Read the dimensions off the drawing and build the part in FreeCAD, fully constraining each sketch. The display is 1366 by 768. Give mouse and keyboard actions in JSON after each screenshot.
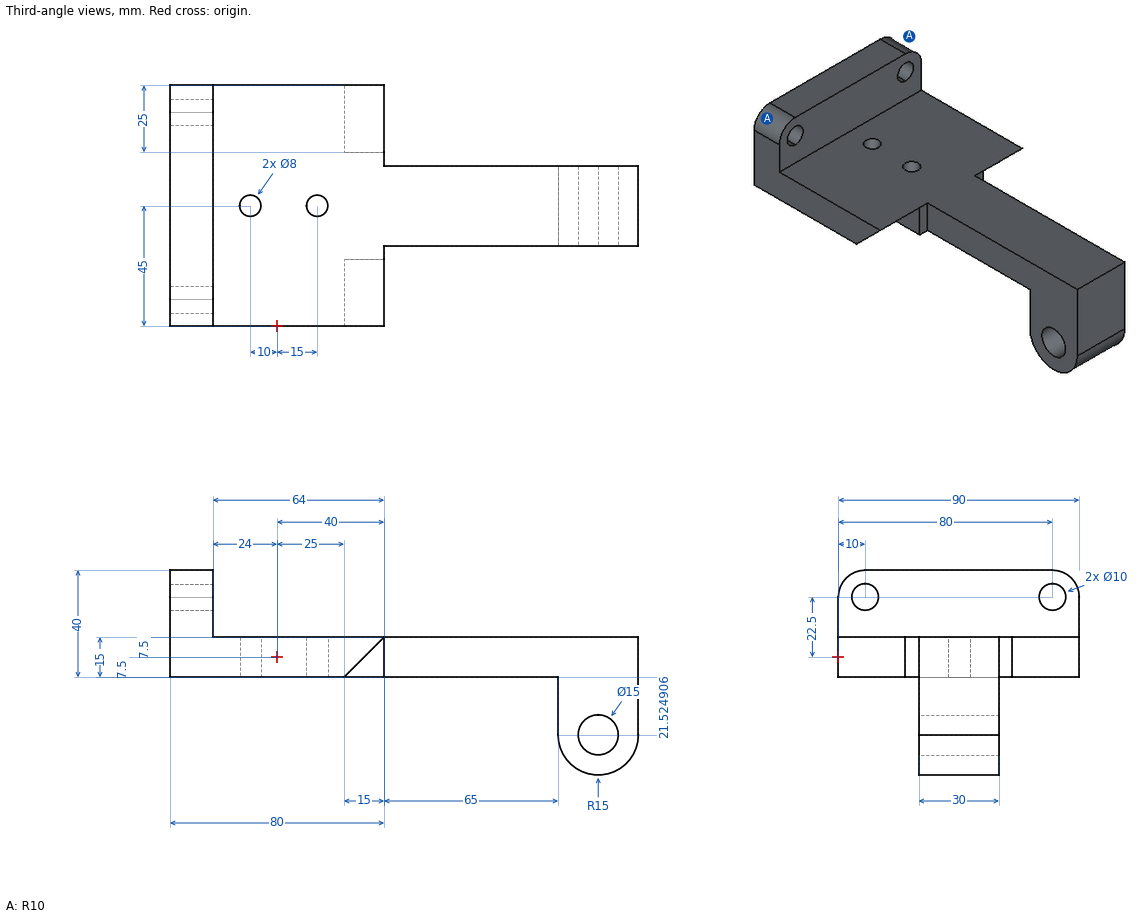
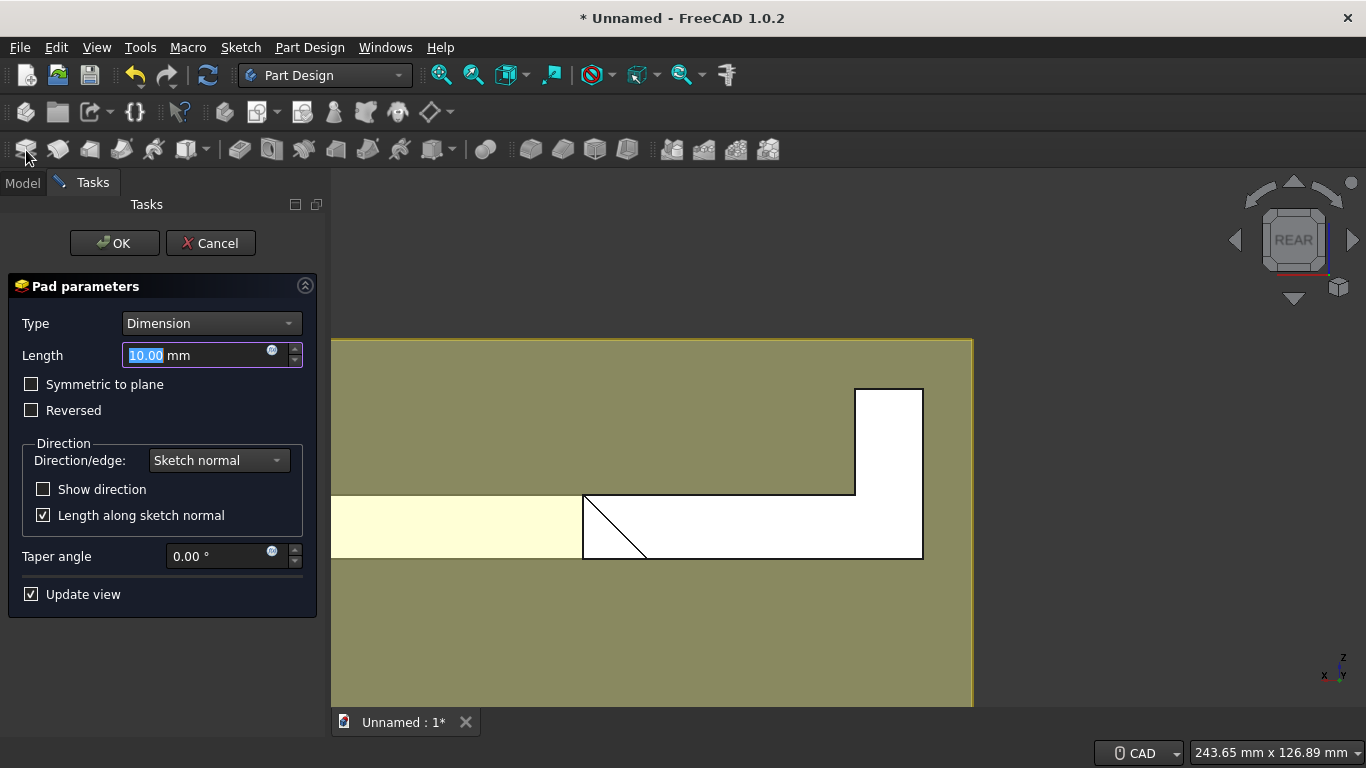
{"action": "type", "text": "30"}
{"action": "key", "text": "Tab"}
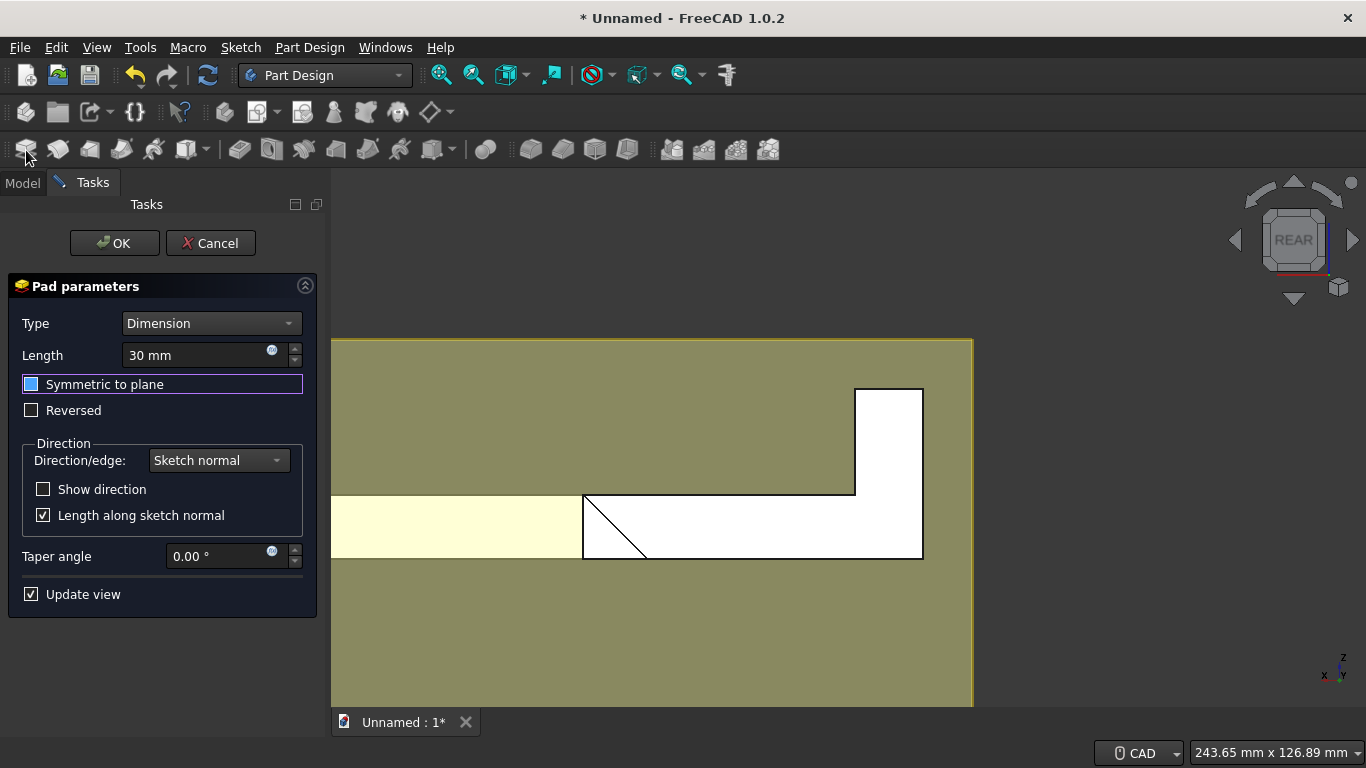
{"action": "left_click", "coordinate": [30, 384]}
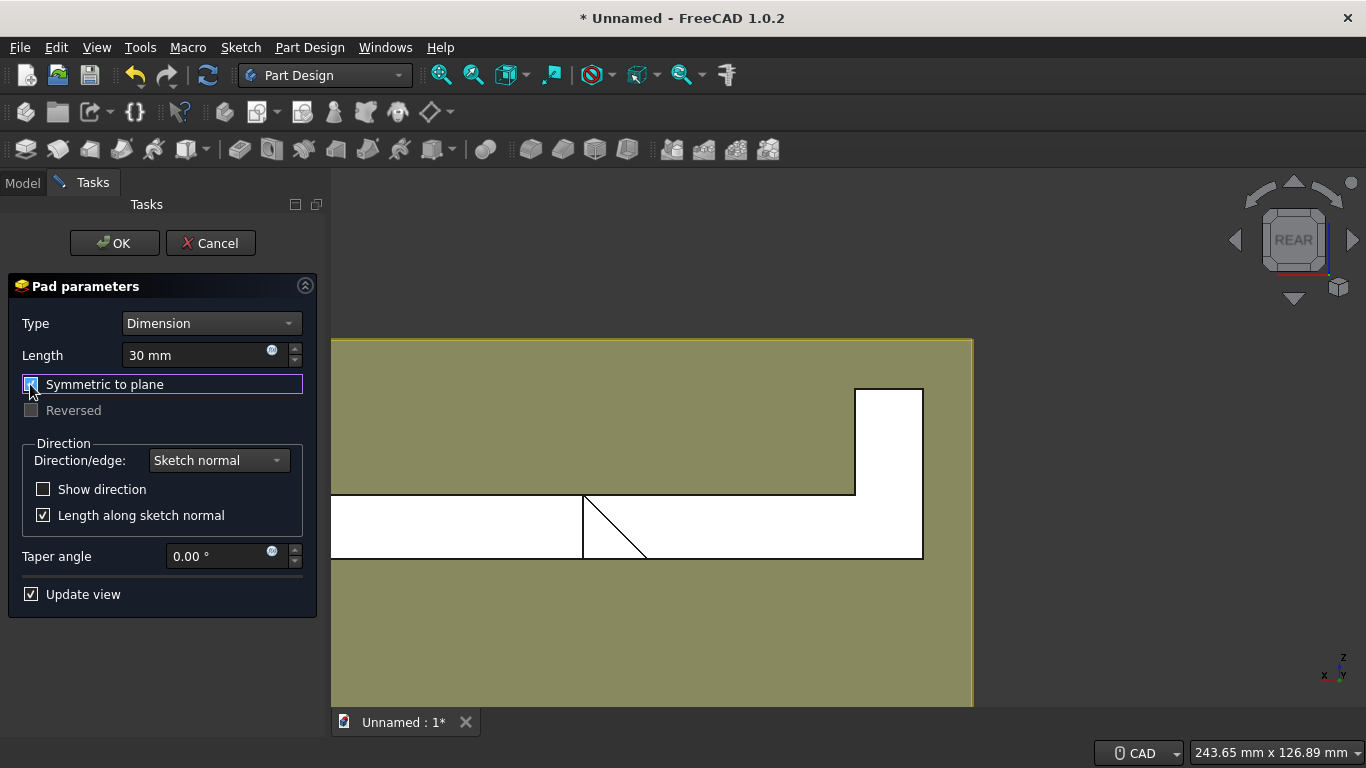
{"action": "left_click", "coordinate": [115, 243]}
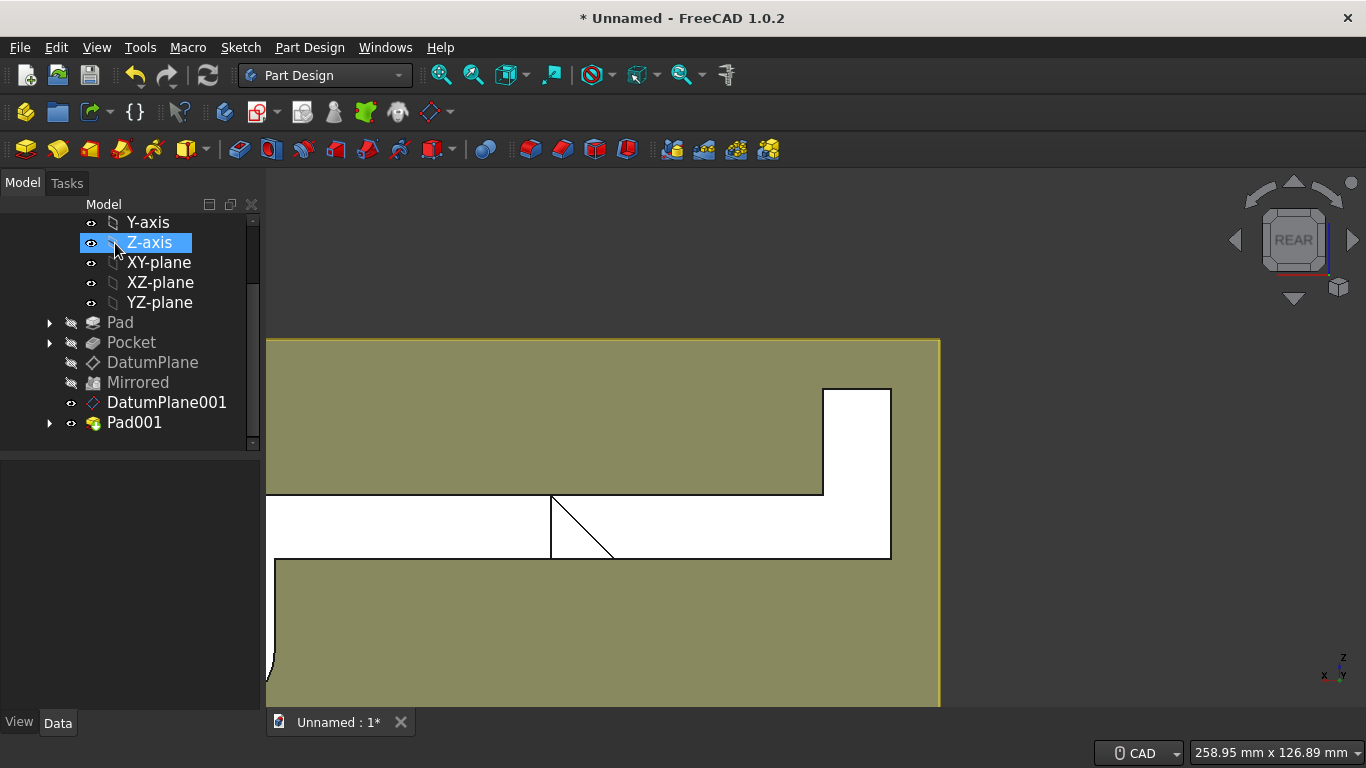
{"action": "left_click", "coordinate": [116, 403]}
{"action": "key", "text": "space"}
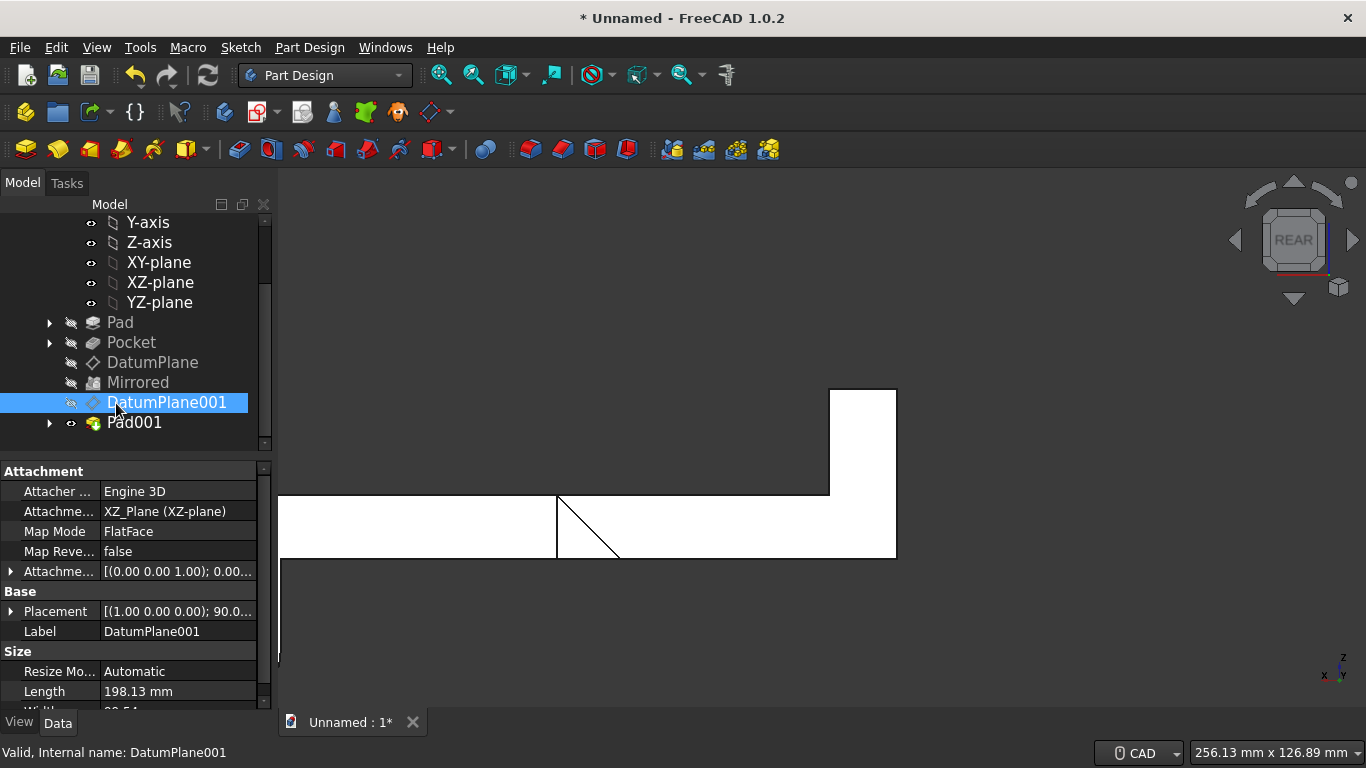
{"action": "left_click", "coordinate": [442, 76]}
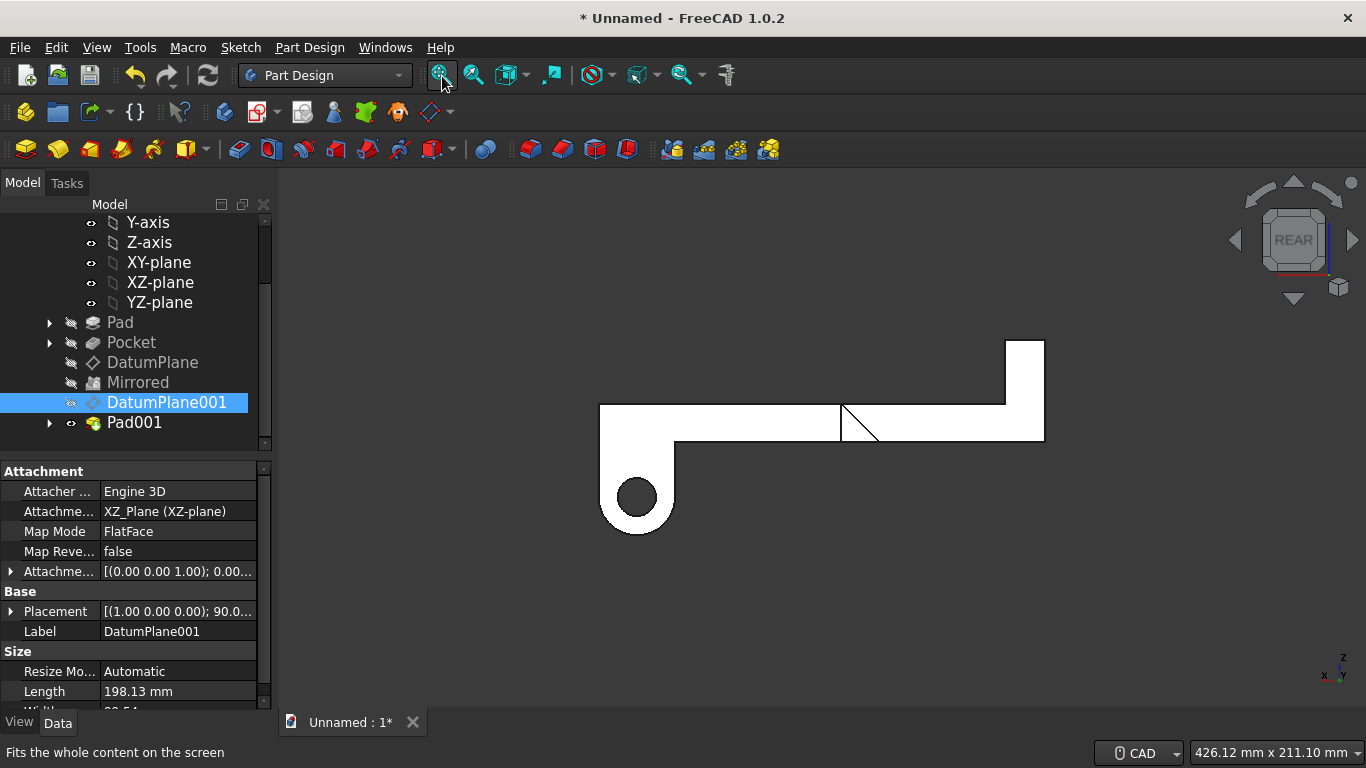
{"action": "key", "text": "0"}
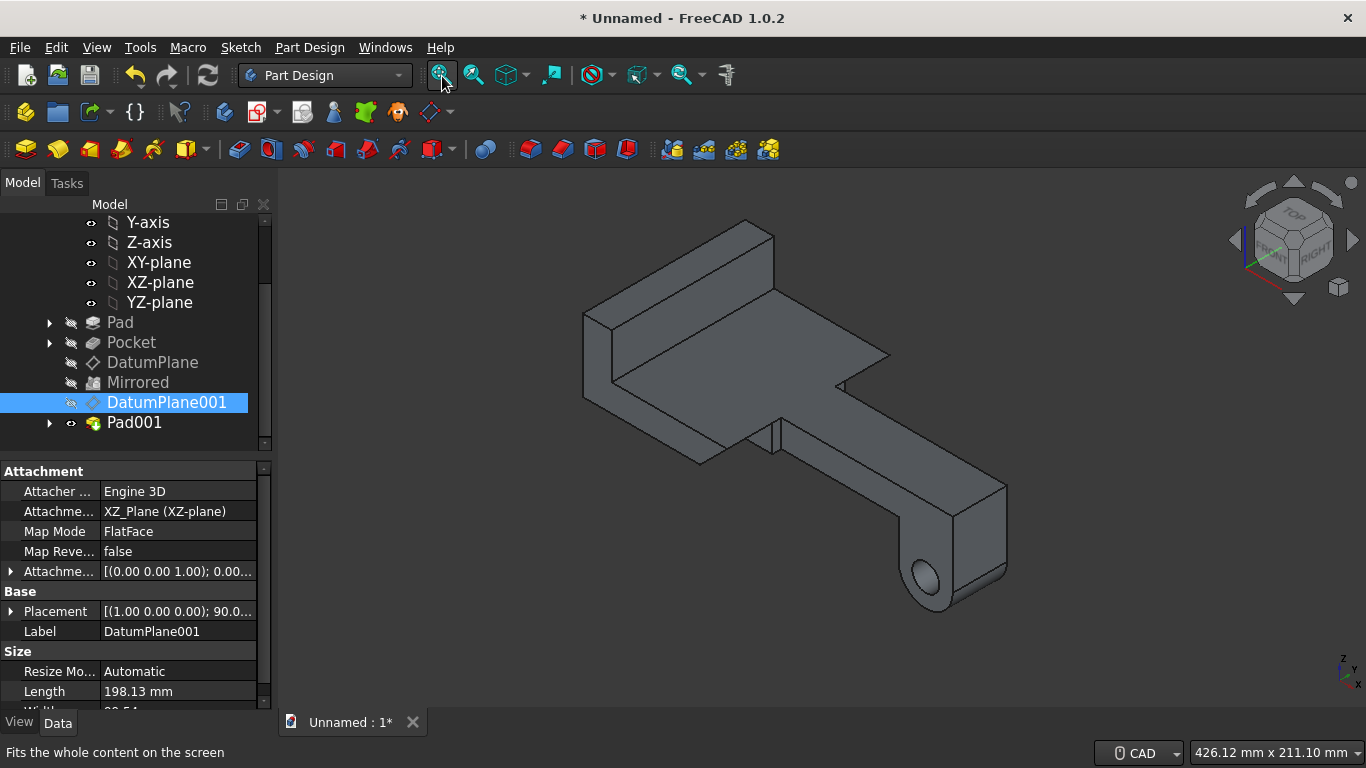
{"action": "left_click", "coordinate": [597, 321]}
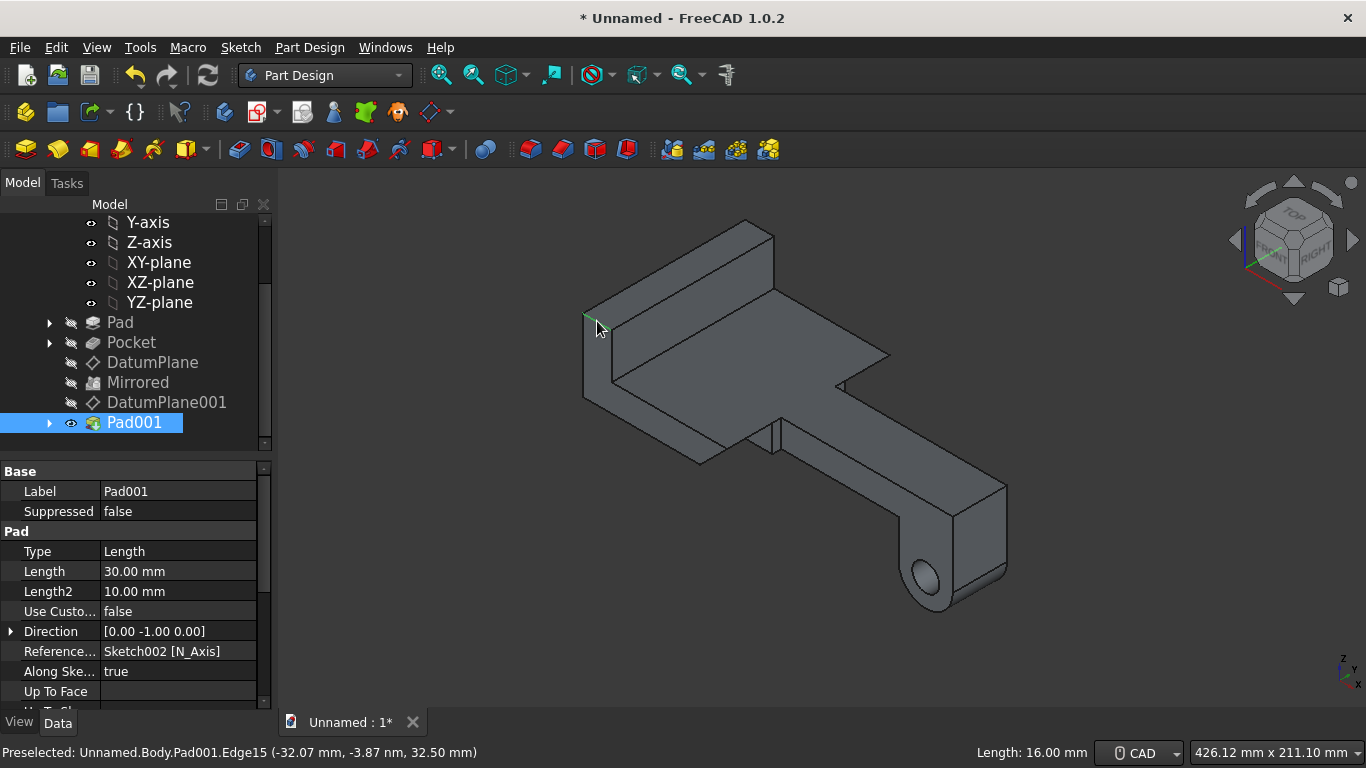
{"action": "key", "text": "2"}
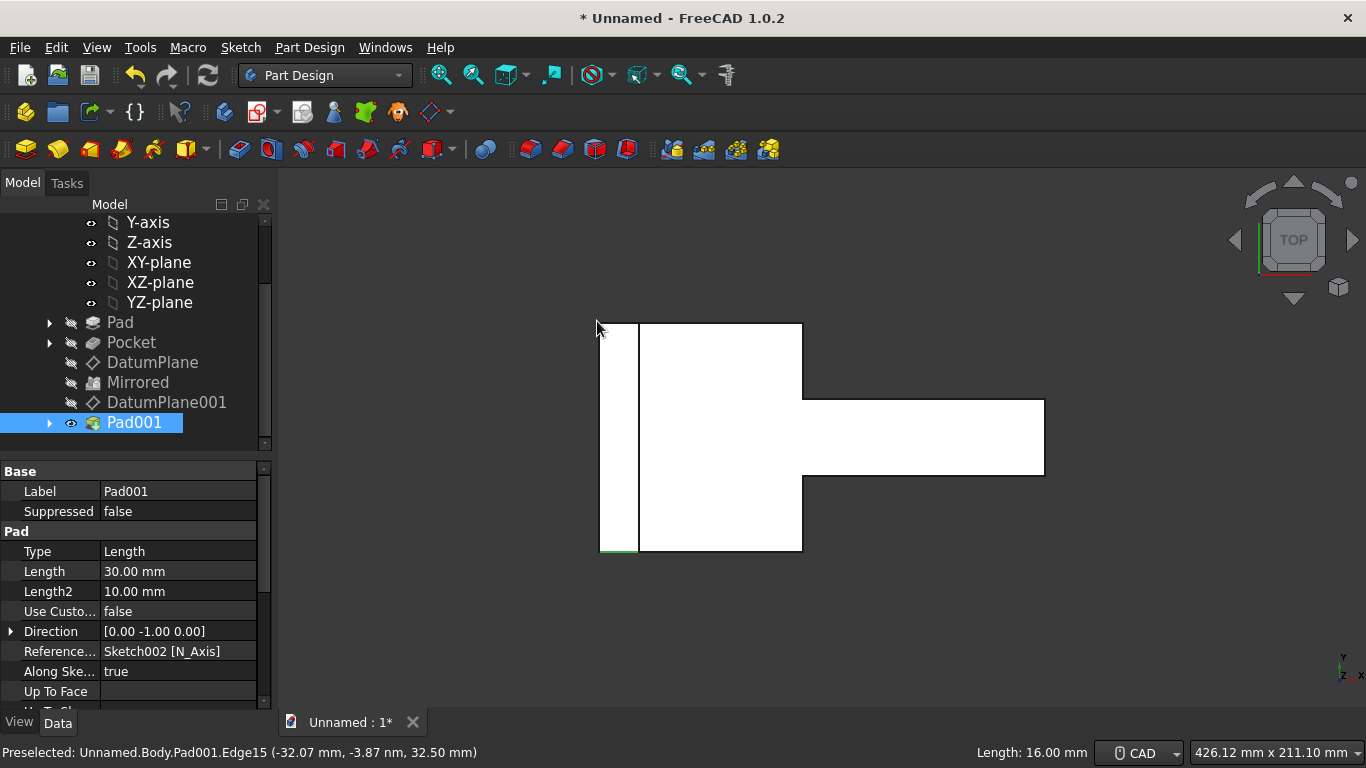
{"action": "left_click", "coordinate": [442, 76]}